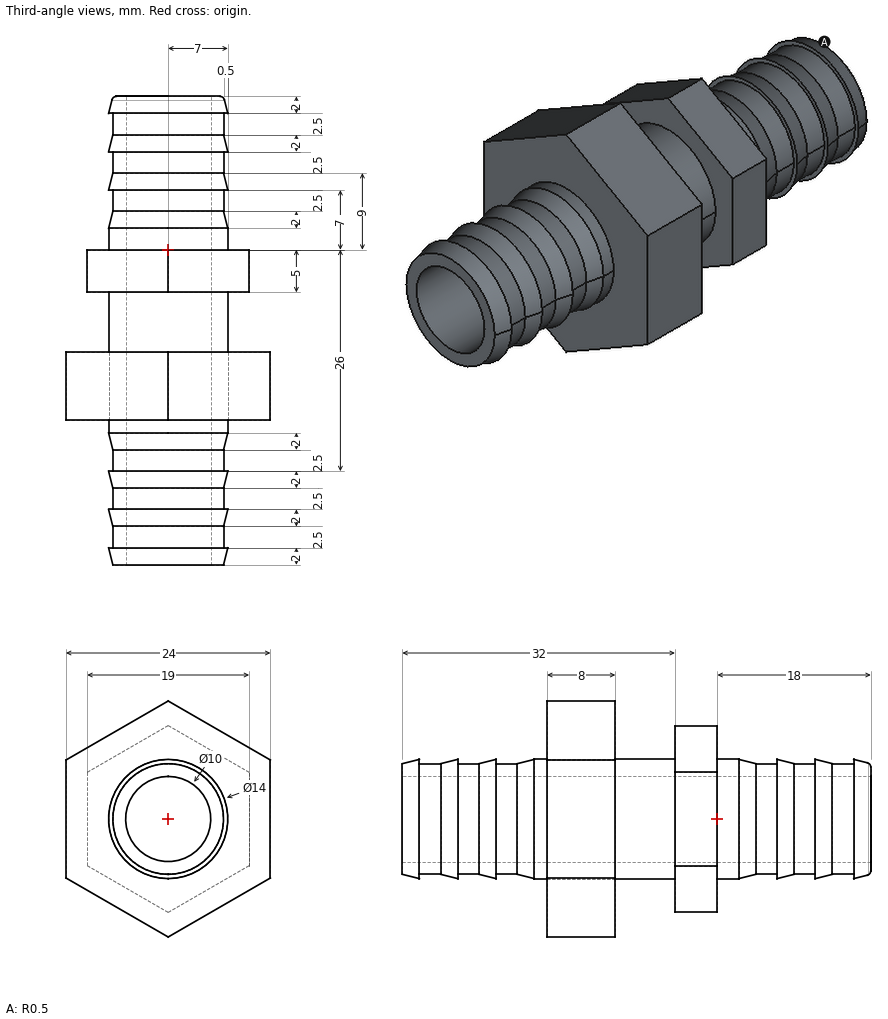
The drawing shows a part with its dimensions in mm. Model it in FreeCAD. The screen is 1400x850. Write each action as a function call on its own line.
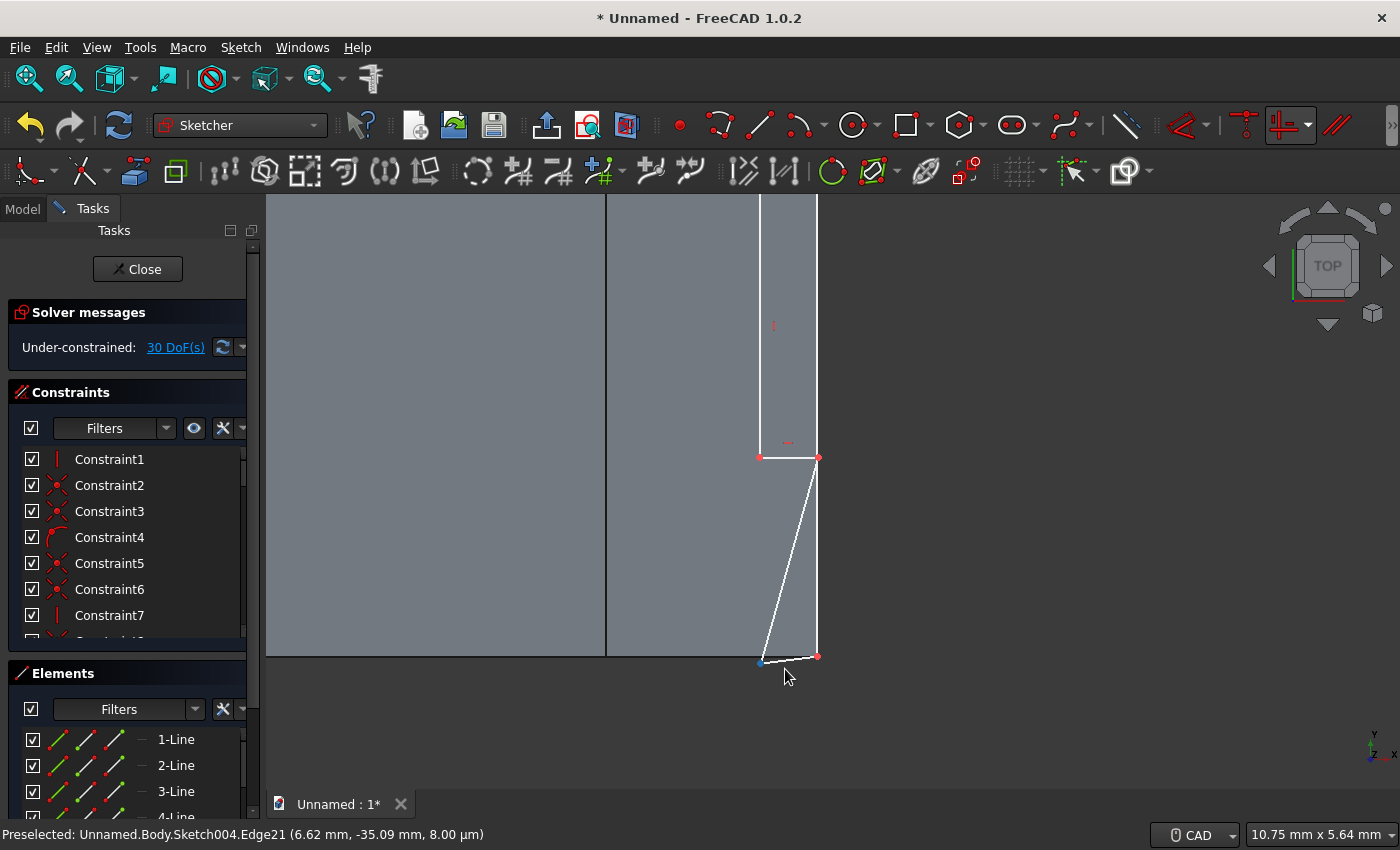
click(778, 662)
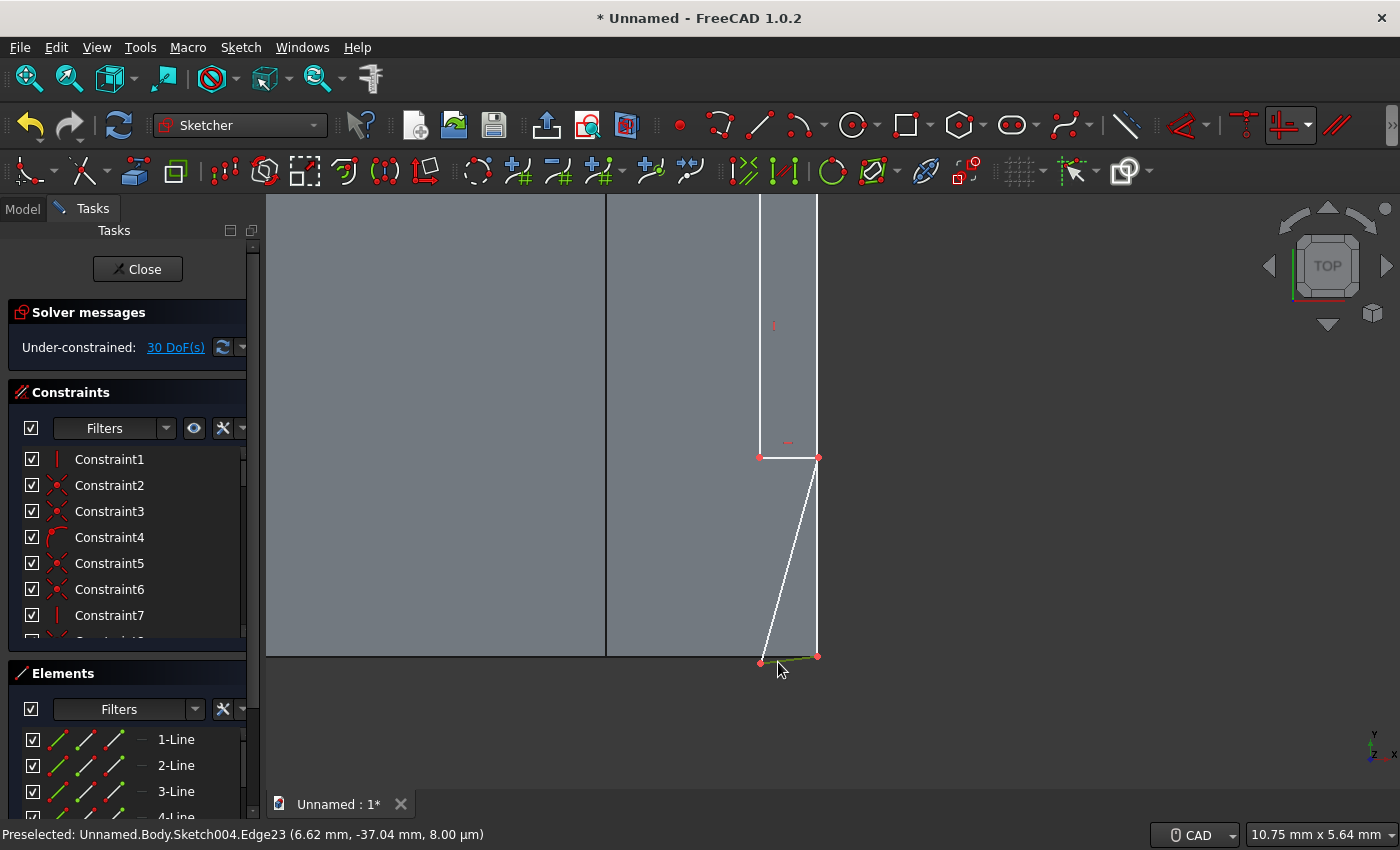
click(1310, 126)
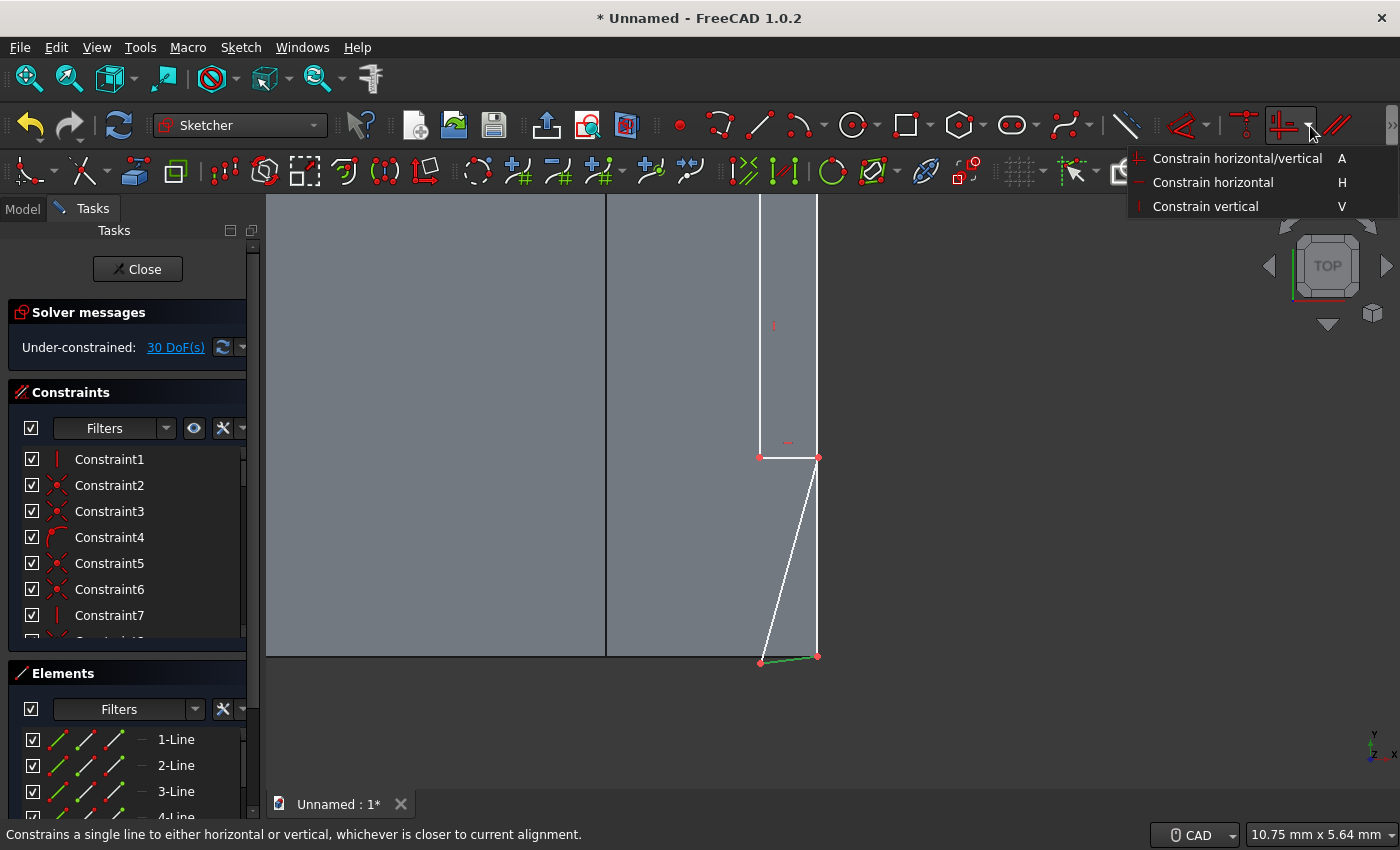
click(1263, 182)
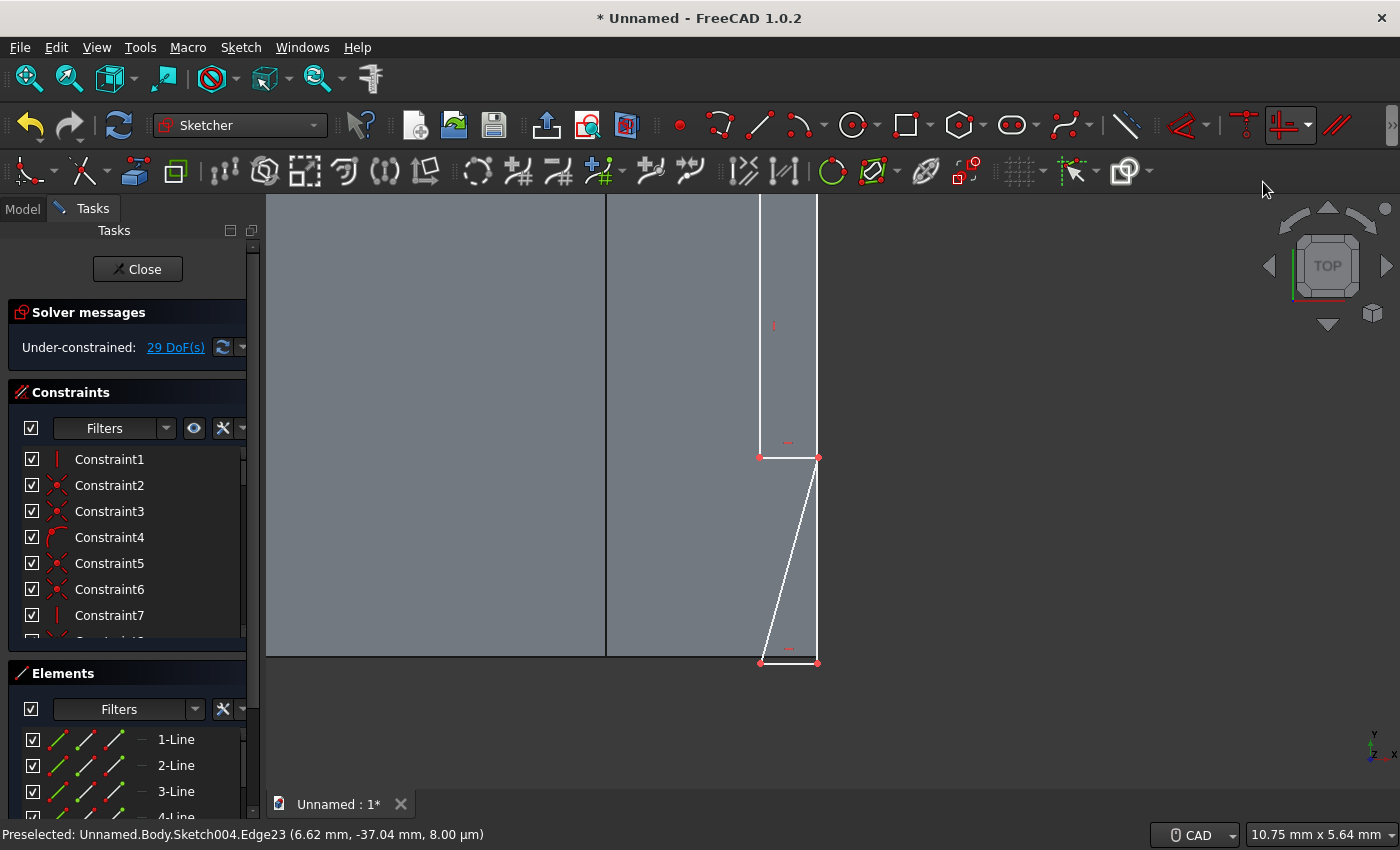
click(1182, 126)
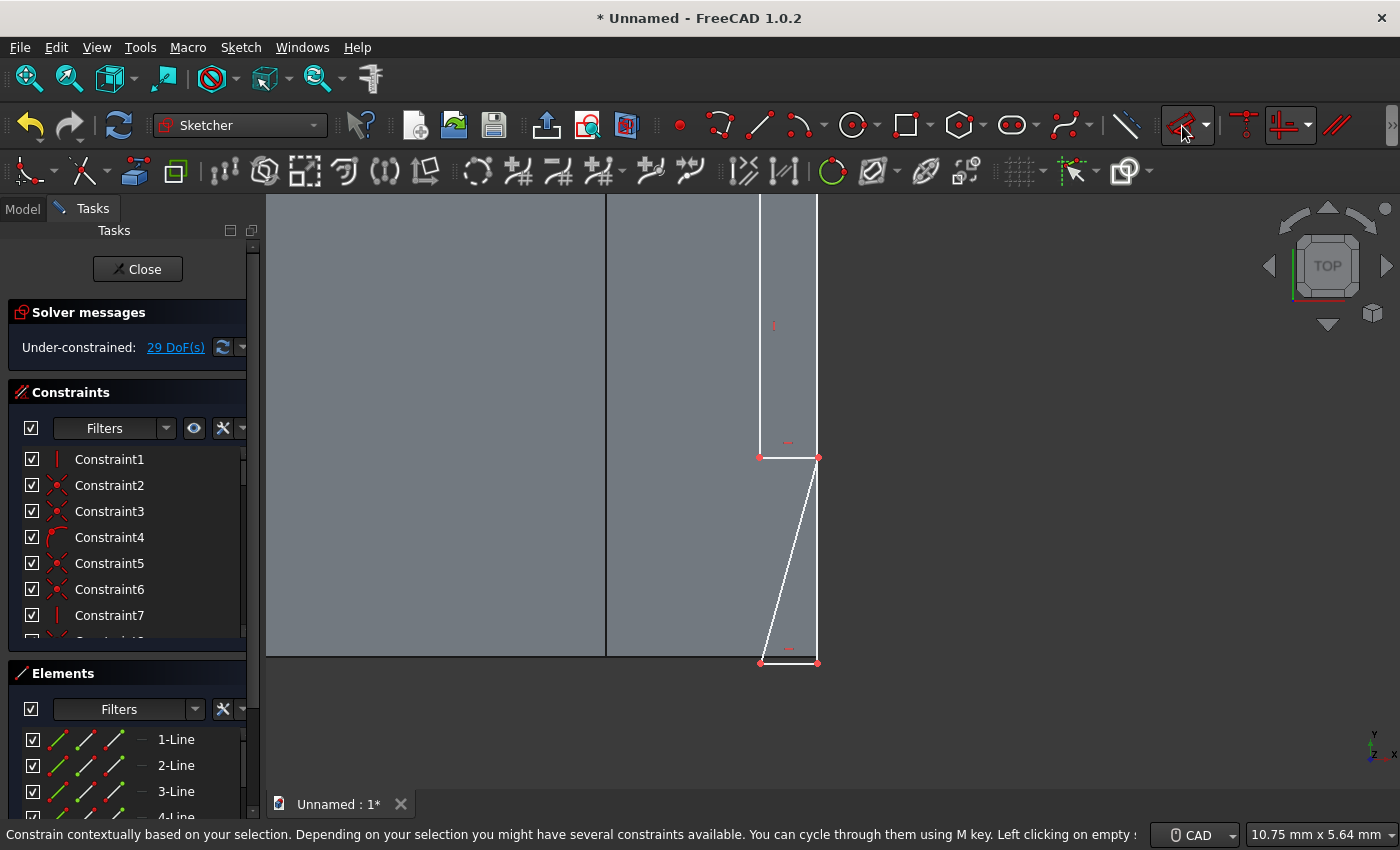
scroll(785, 669, down, 14)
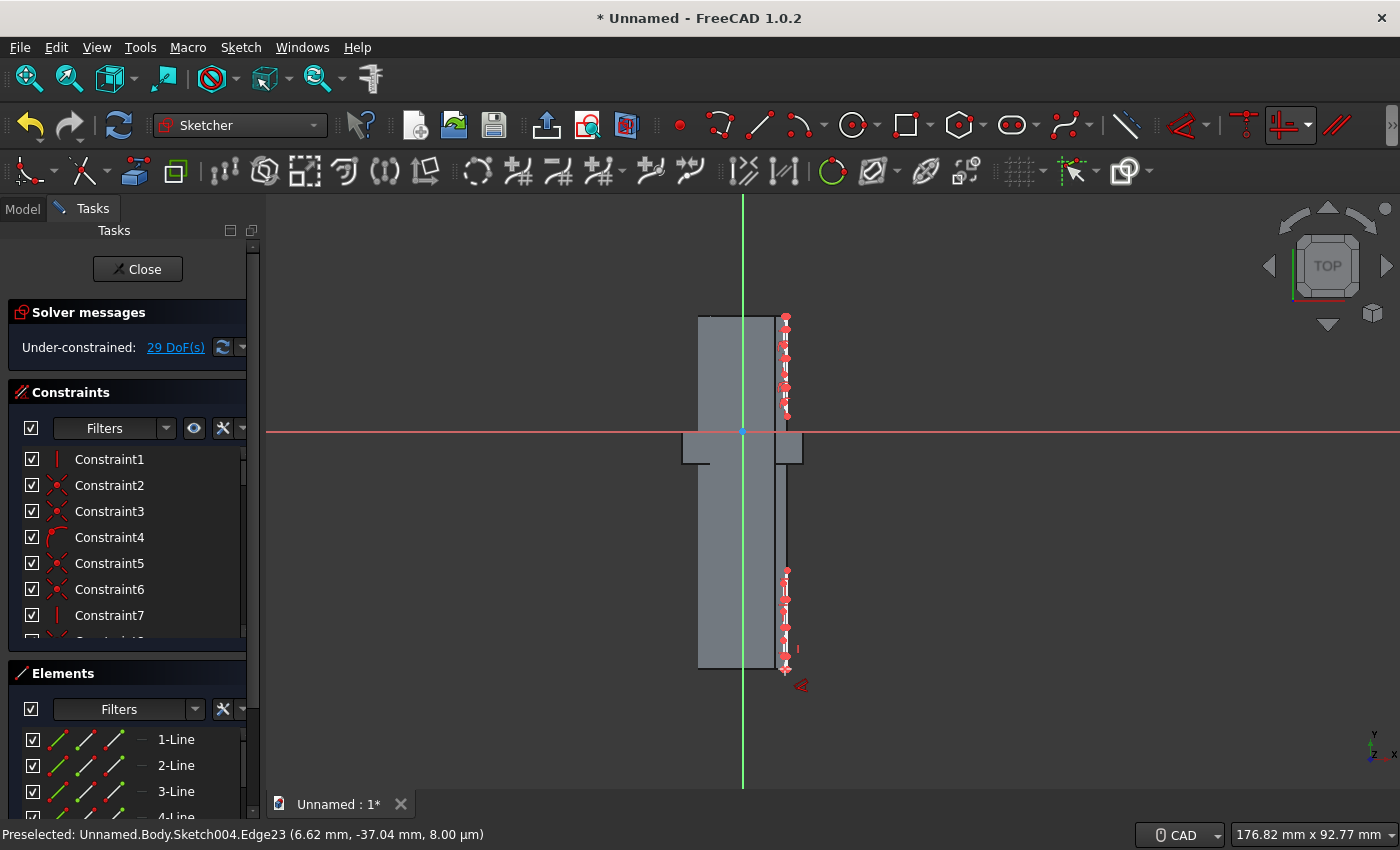
click(787, 417)
click(765, 383)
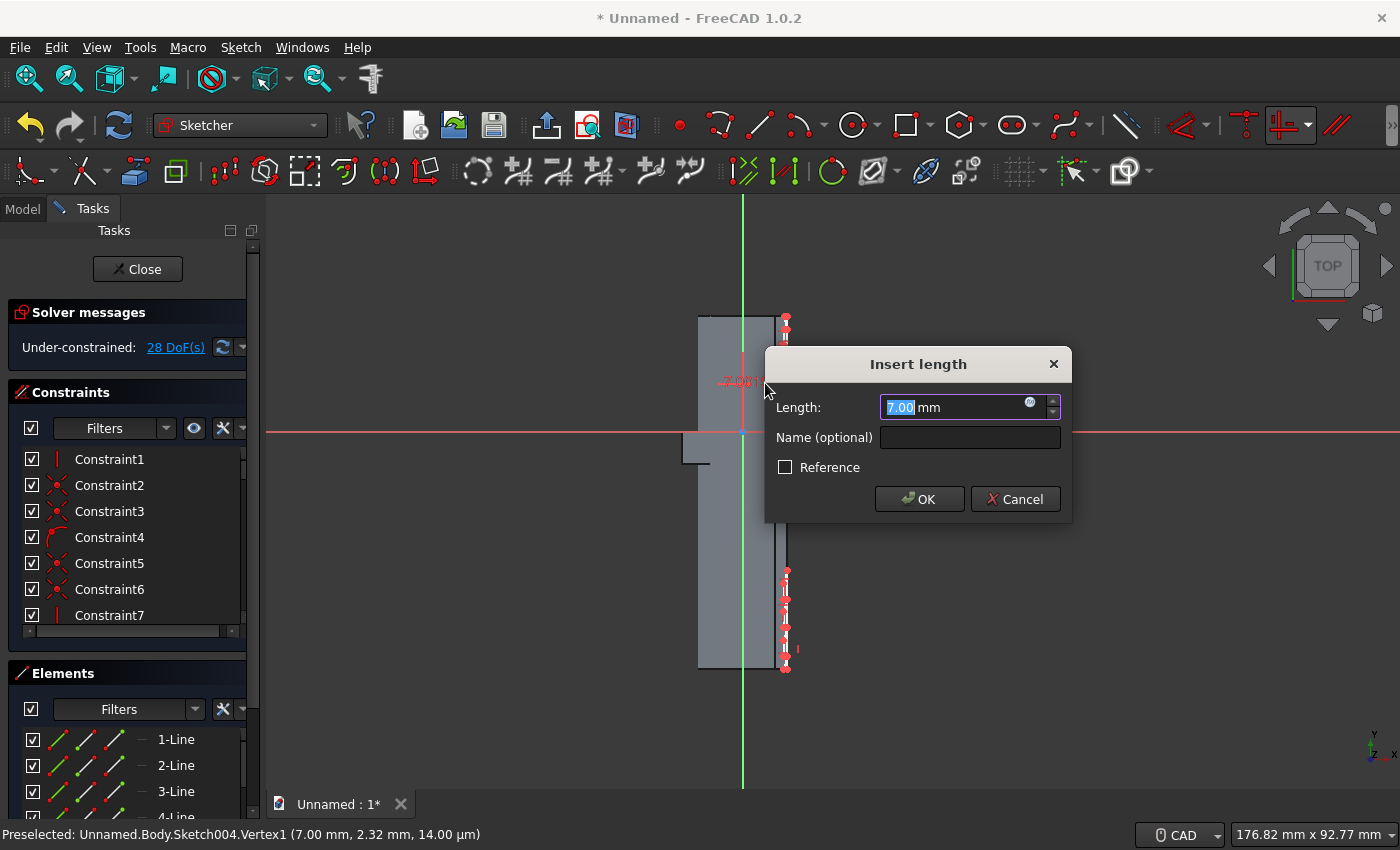
text(7)
key(Return)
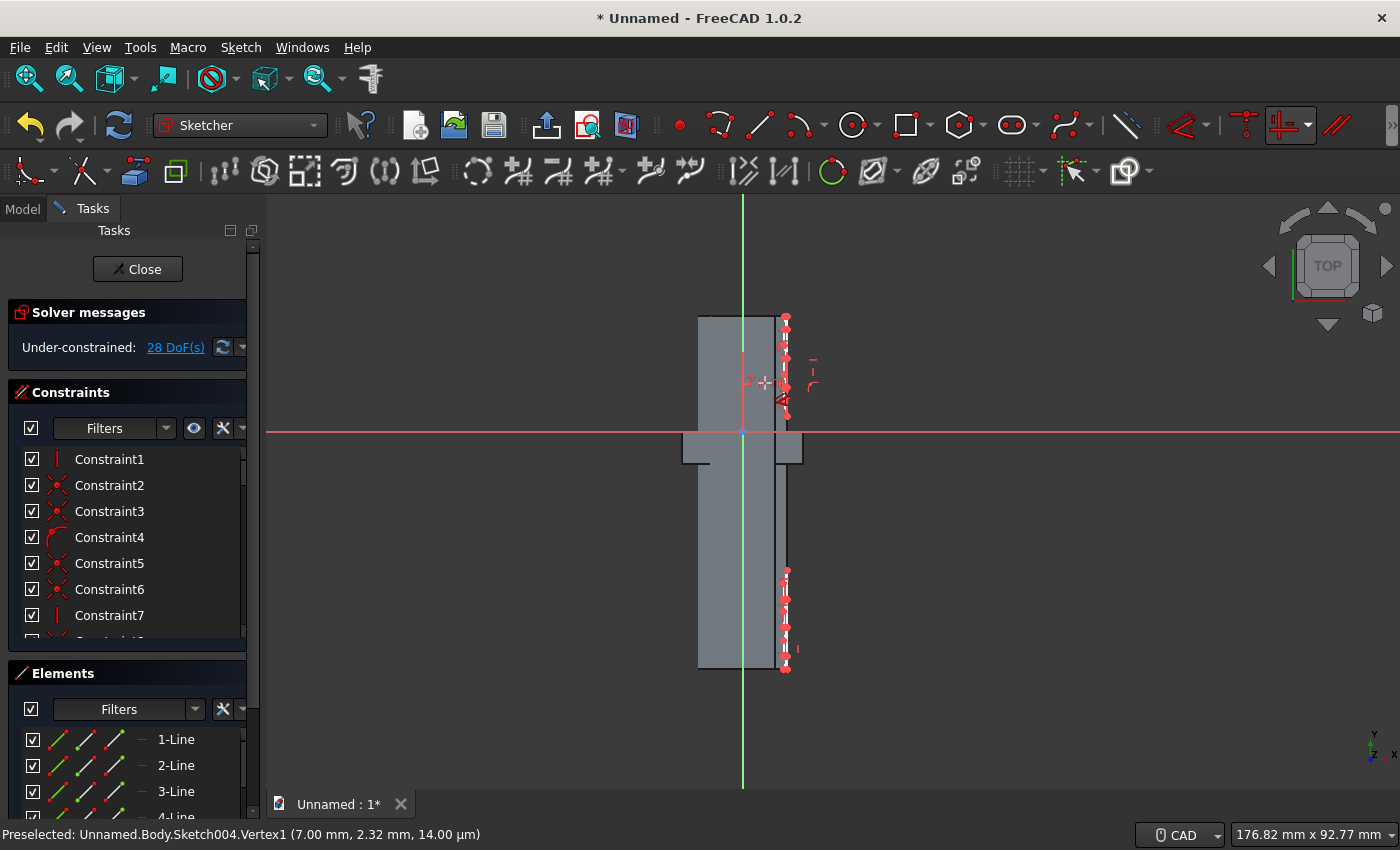
click(784, 374)
click(709, 403)